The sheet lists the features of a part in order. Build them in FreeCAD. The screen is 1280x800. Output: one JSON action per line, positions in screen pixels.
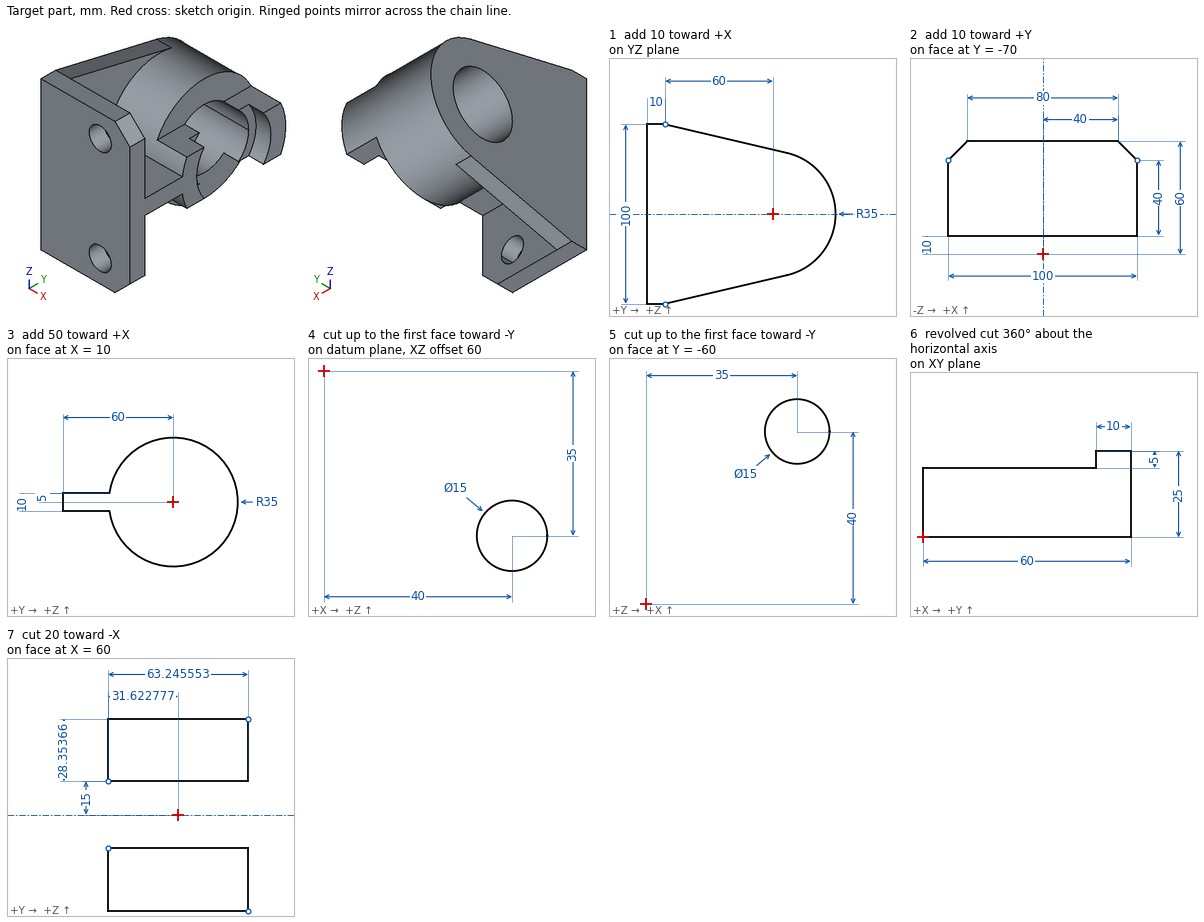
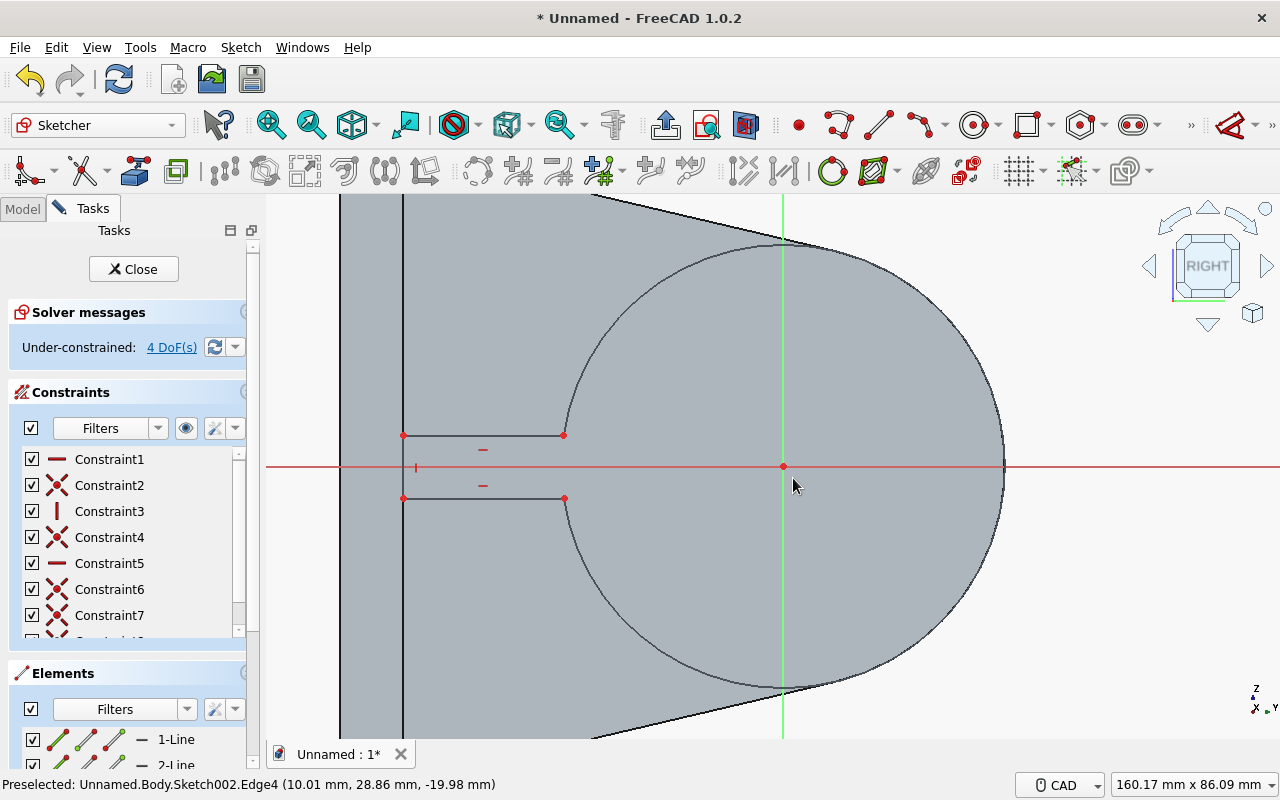
{"action": "key", "text": "d"}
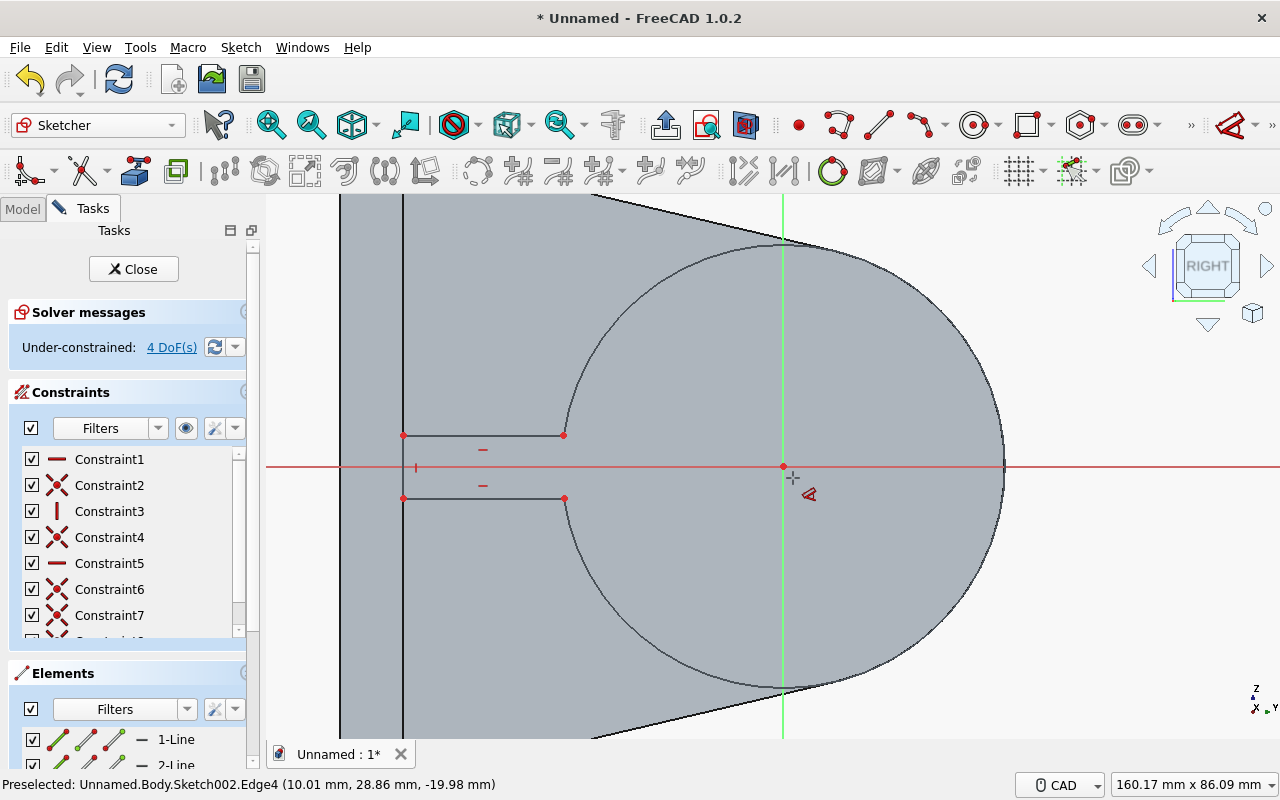
{"action": "left_click", "coordinate": [865, 673]}
{"action": "left_click", "coordinate": [877, 703]}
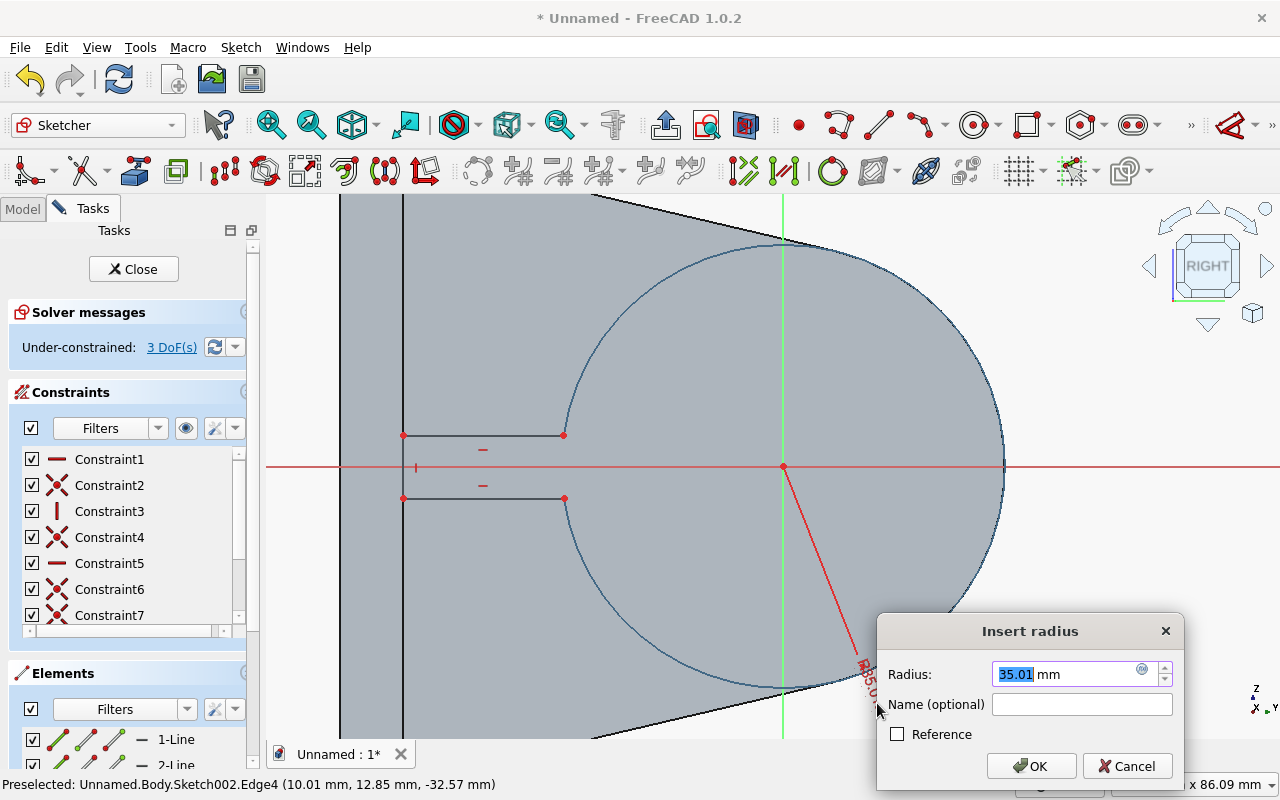
{"action": "type", "text": "35"}
{"action": "key", "text": "Return"}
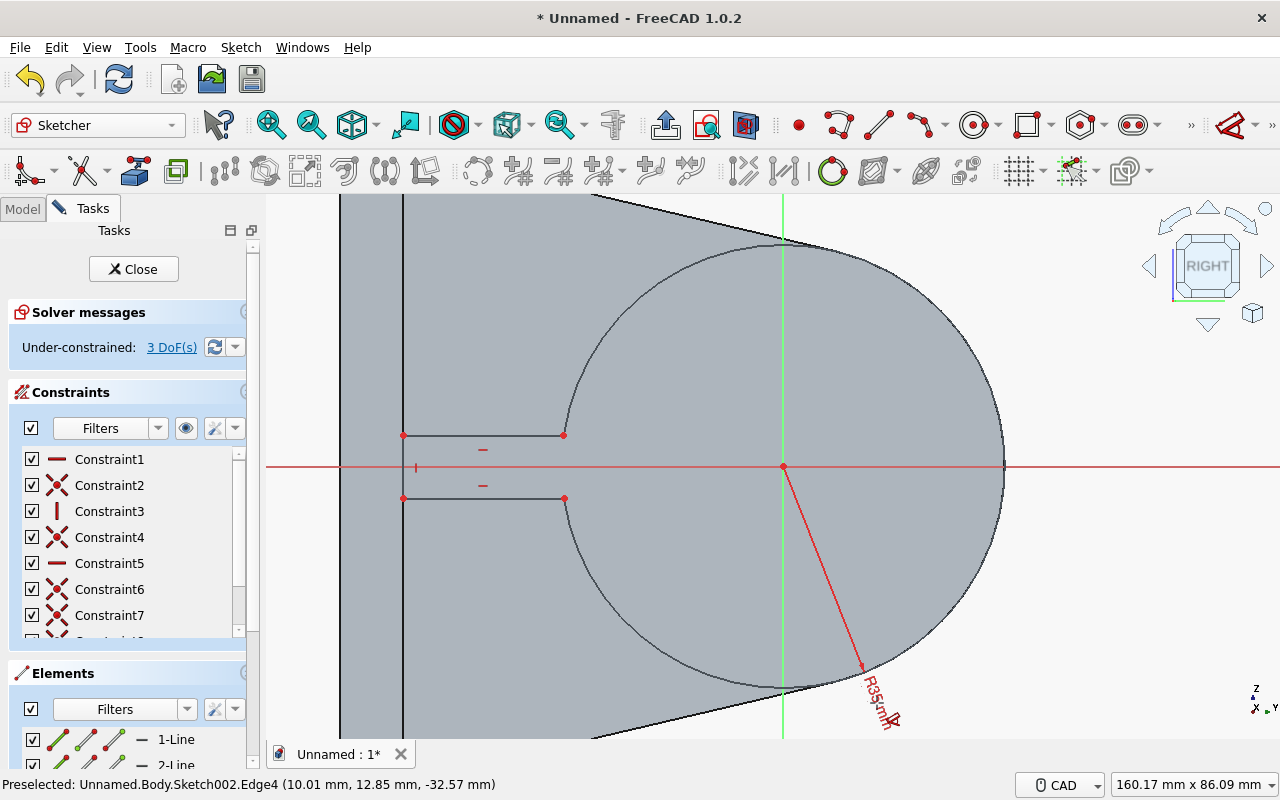
{"action": "left_click", "coordinate": [403, 455]}
{"action": "left_click", "coordinate": [369, 453]}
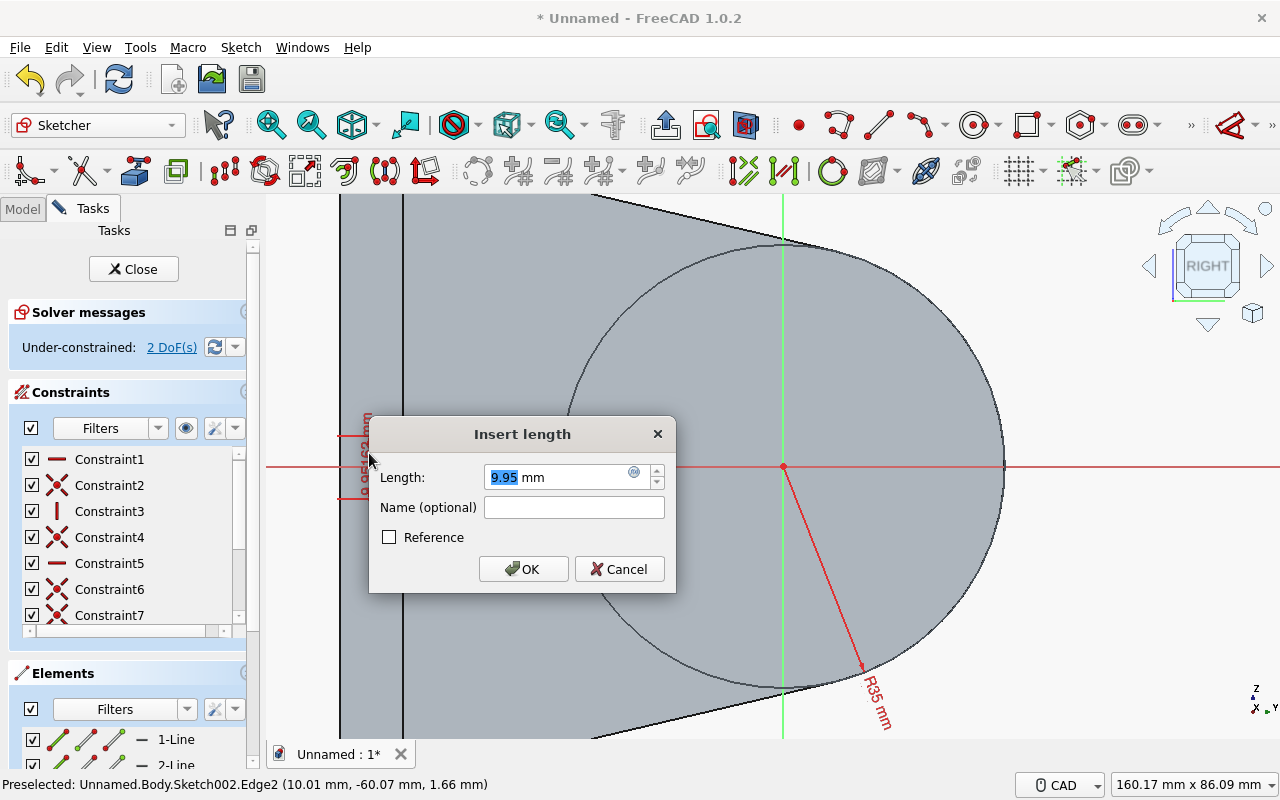
{"action": "type", "text": "10"}
{"action": "key", "text": "Return"}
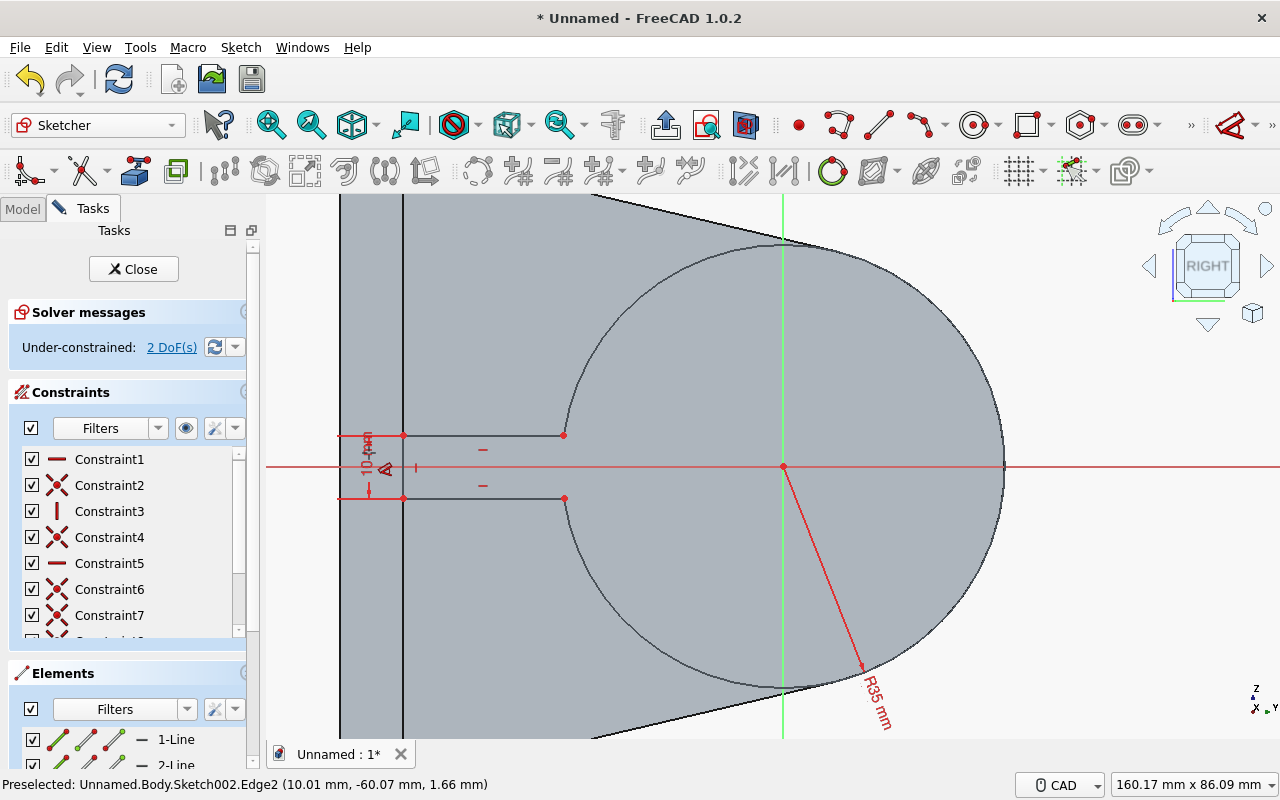
{"action": "scroll", "coordinate": [564, 436], "scroll_direction": "up", "scroll_amount": 2}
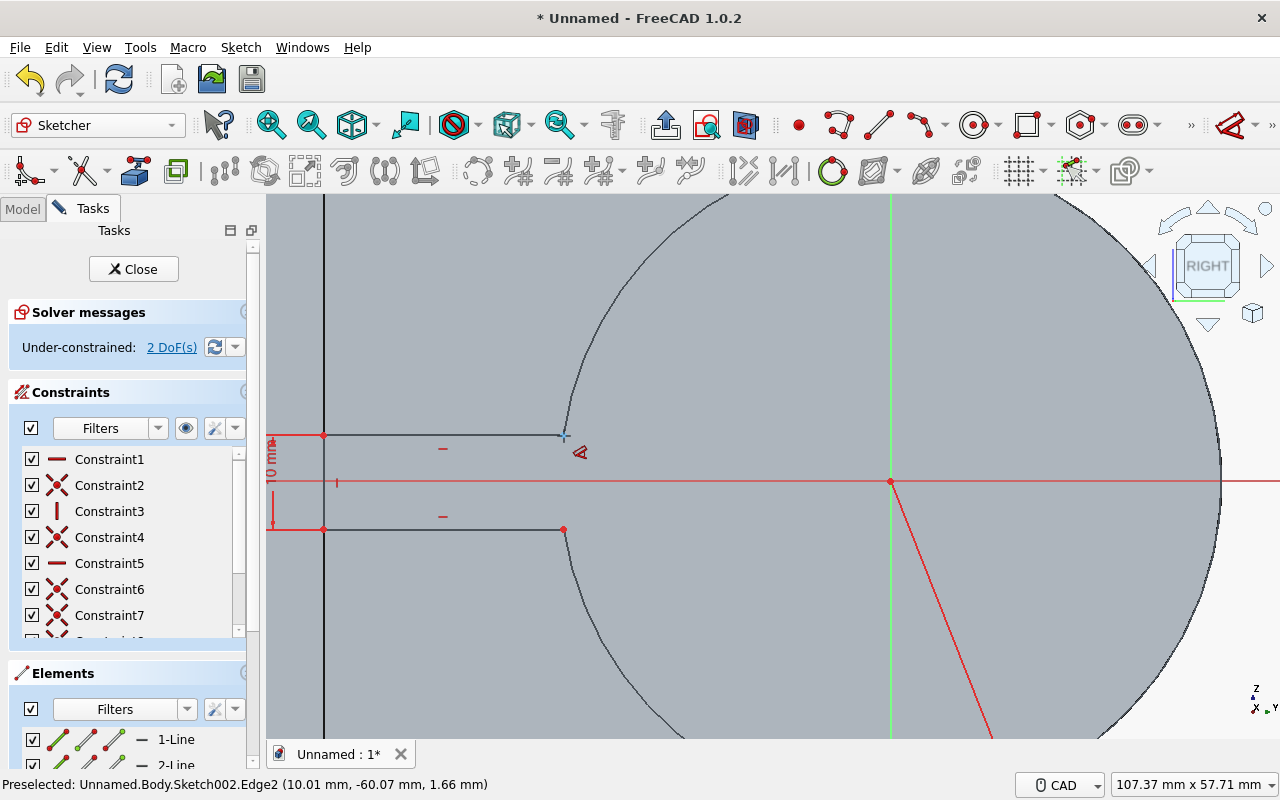
{"action": "left_click", "coordinate": [564, 435]}
{"action": "left_click", "coordinate": [530, 458]}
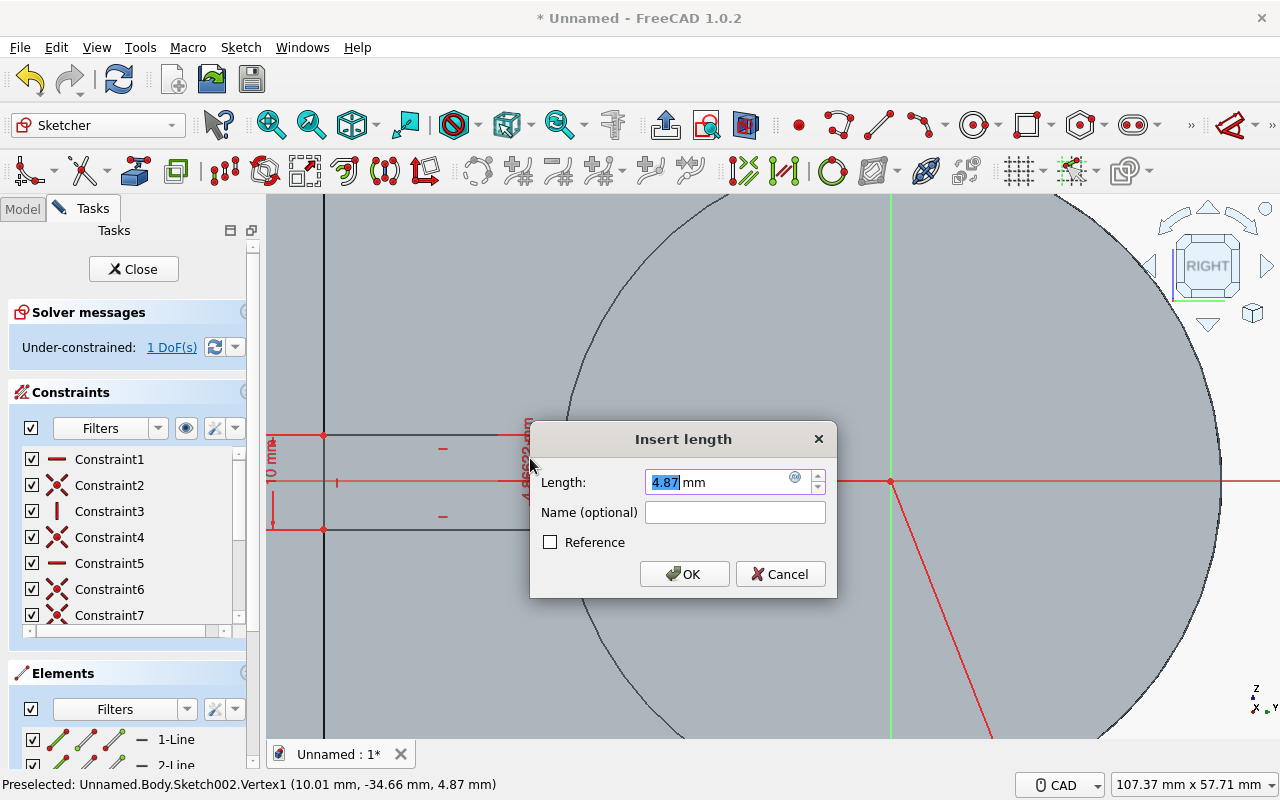
{"action": "type", "text": "5"}
{"action": "key", "text": "Return"}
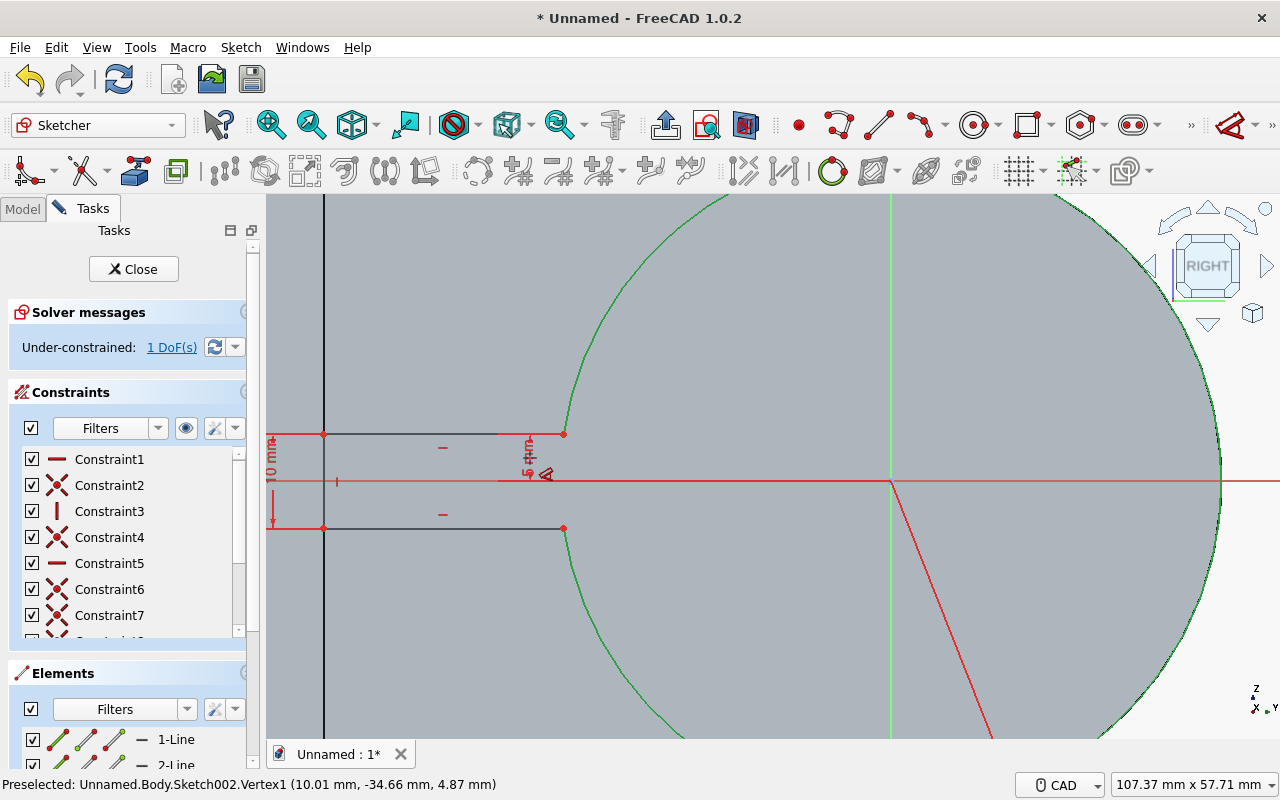
{"action": "left_click", "coordinate": [324, 434]}
{"action": "left_click", "coordinate": [607, 400]}